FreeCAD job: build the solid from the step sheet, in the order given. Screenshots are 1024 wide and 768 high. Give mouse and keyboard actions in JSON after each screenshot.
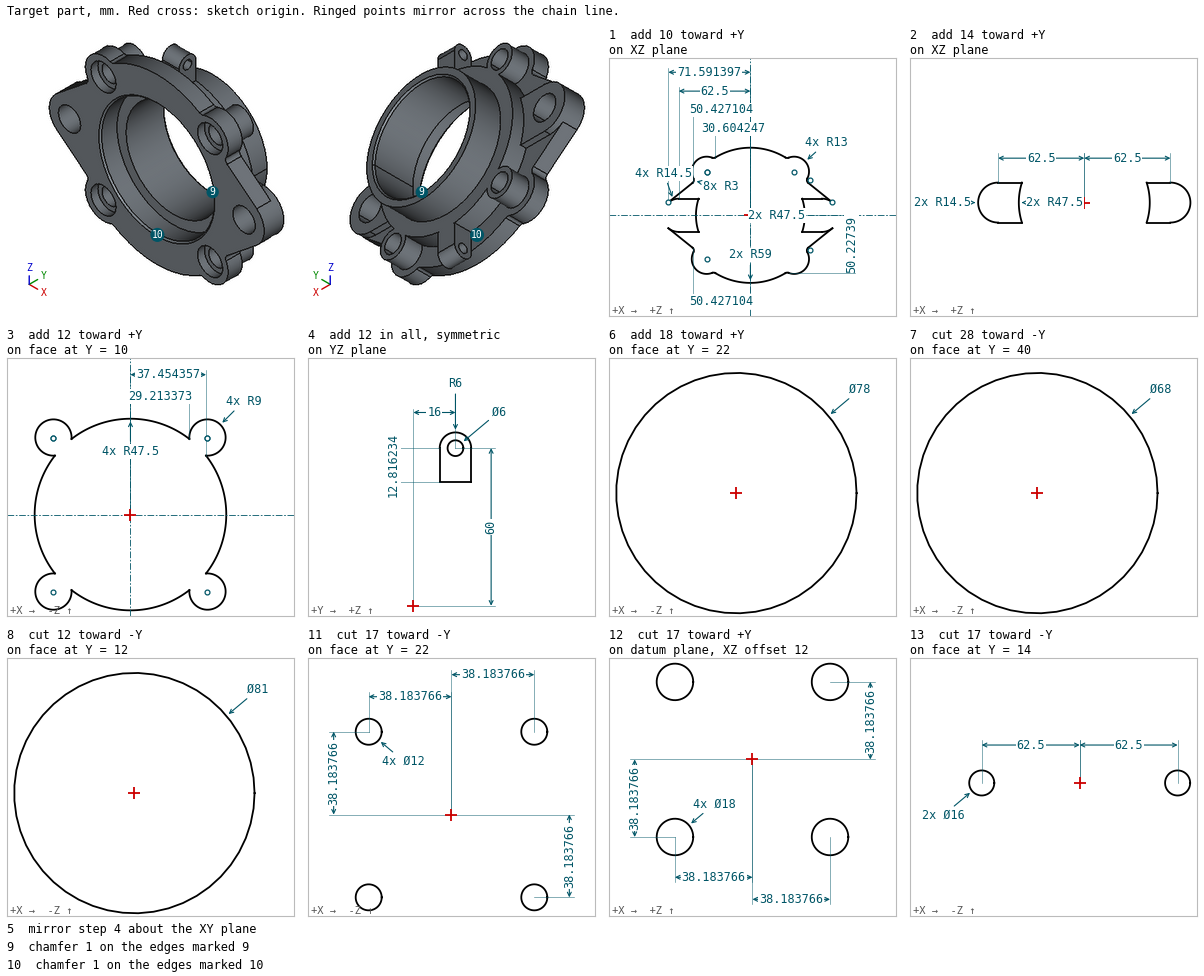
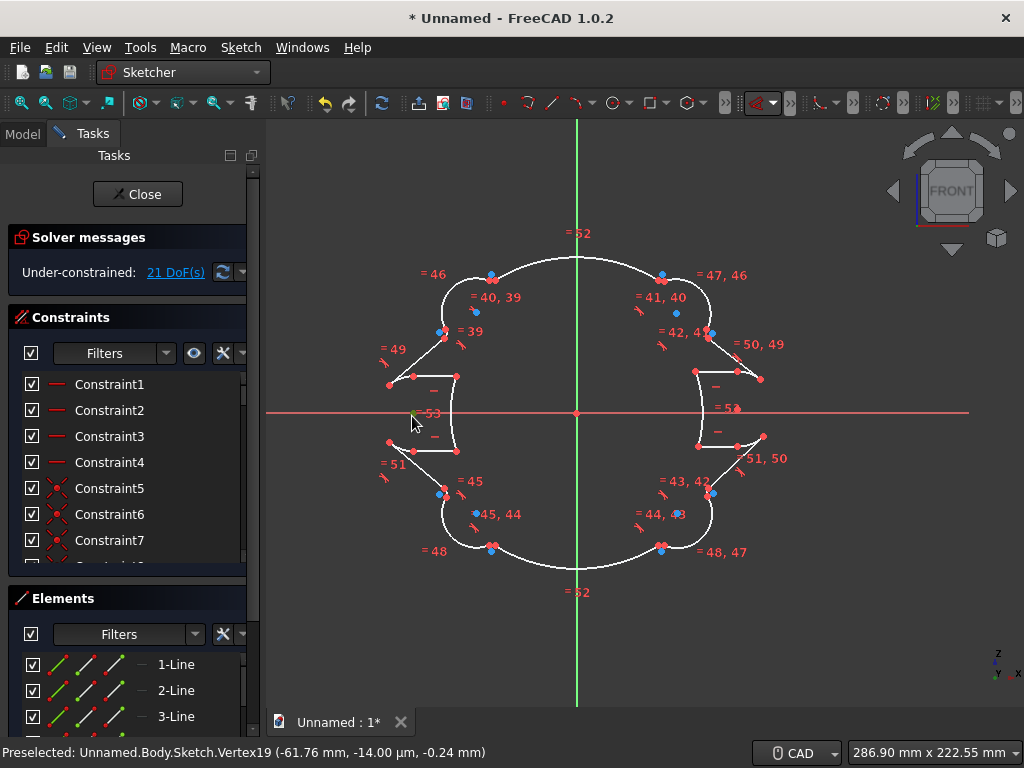
{"action": "left_click", "coordinate": [334, 413]}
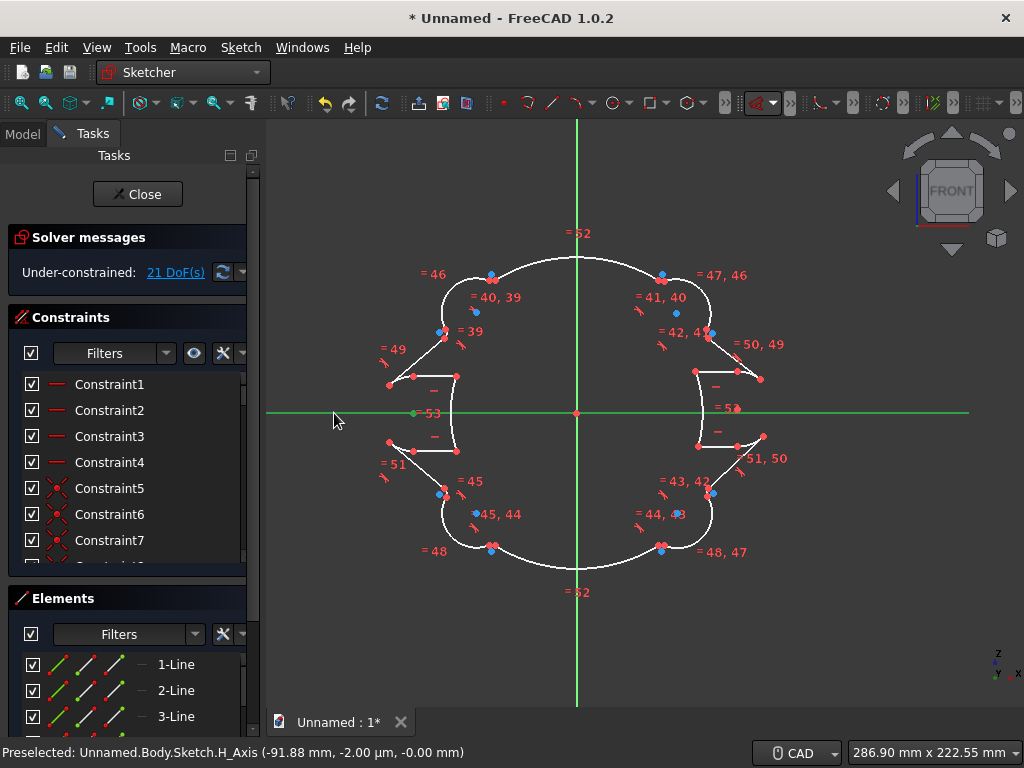
{"action": "key", "text": "c"}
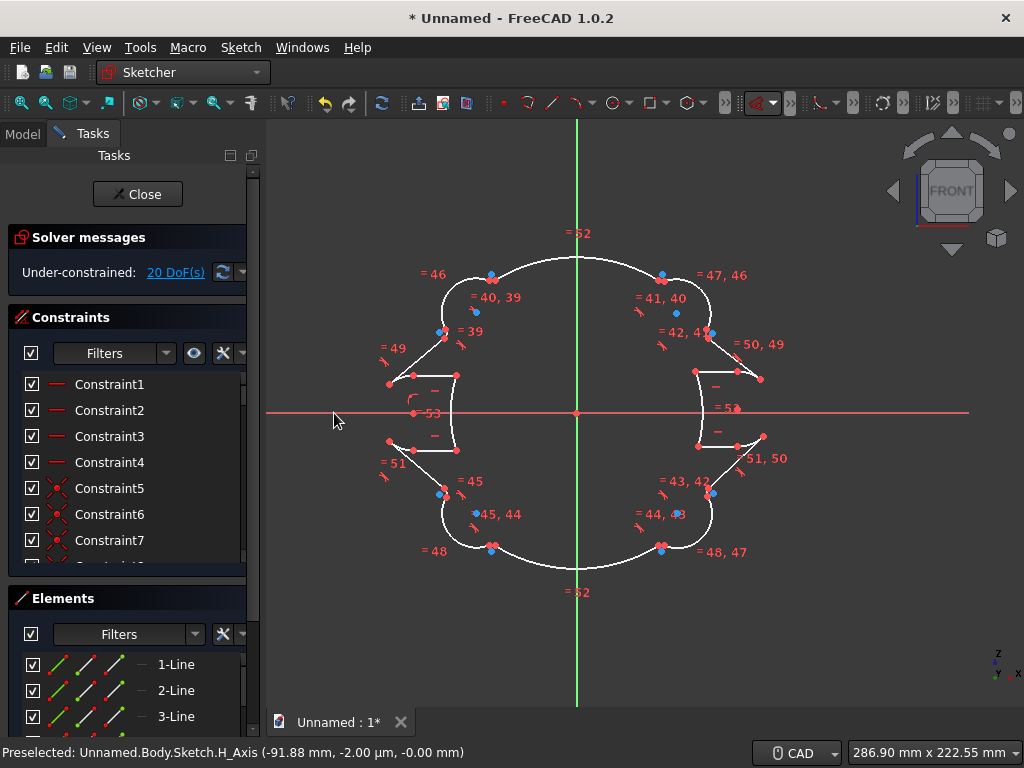
{"action": "left_click", "coordinate": [738, 409]}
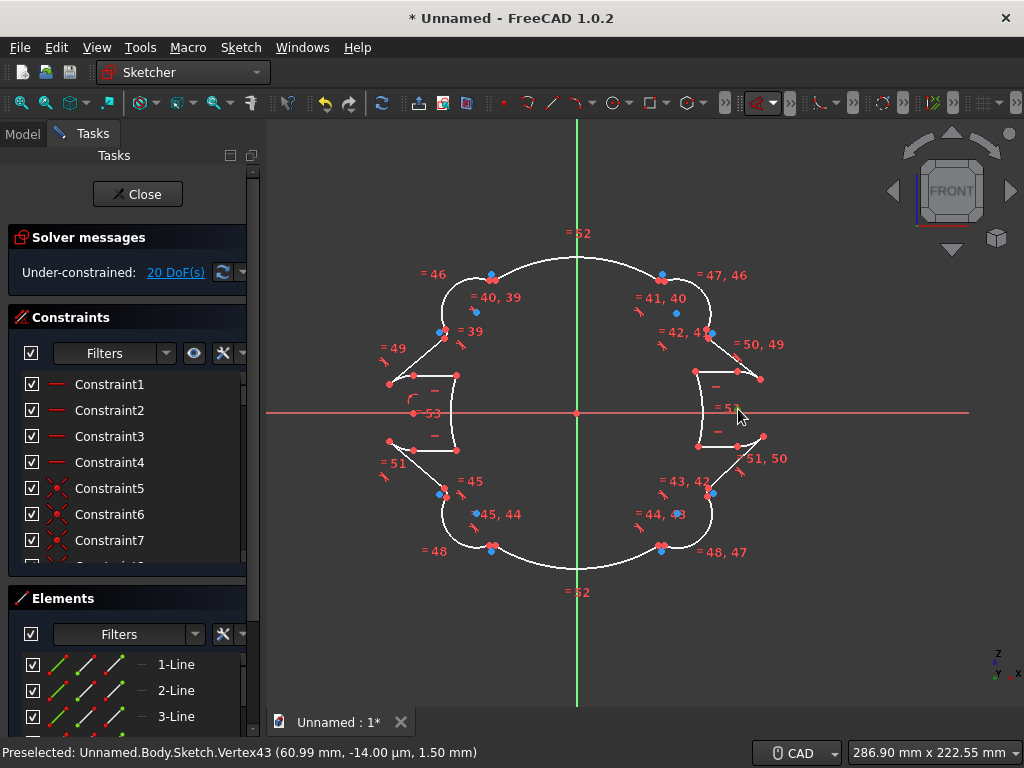
{"action": "left_click", "coordinate": [334, 413]}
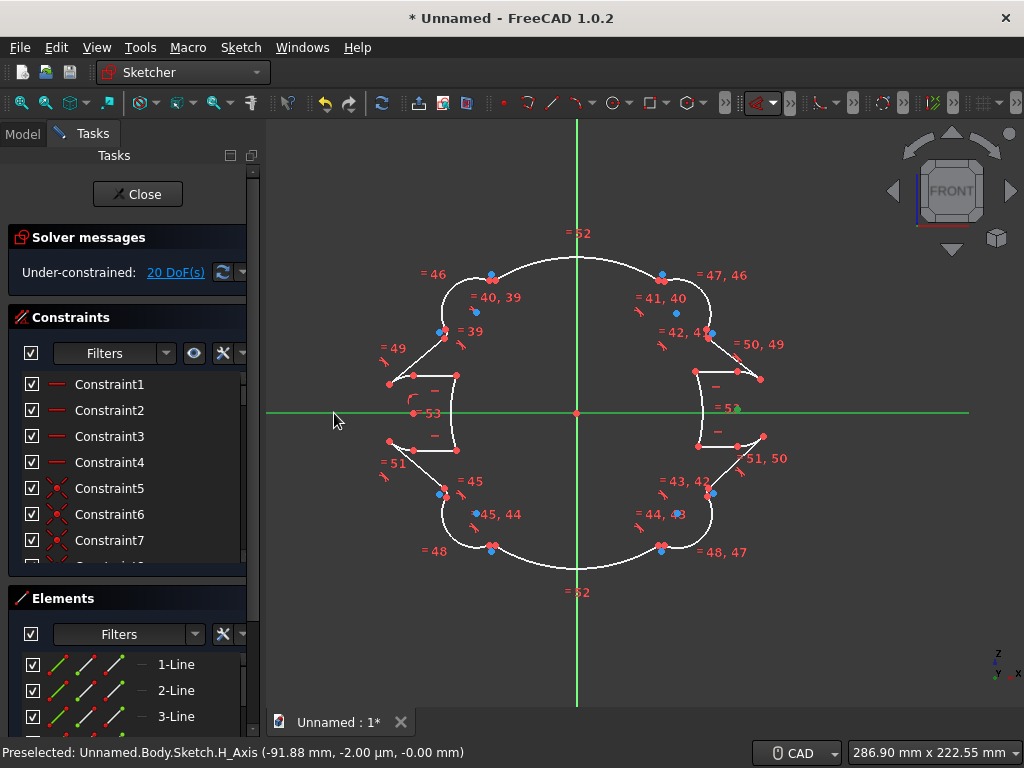
{"action": "key", "text": "c"}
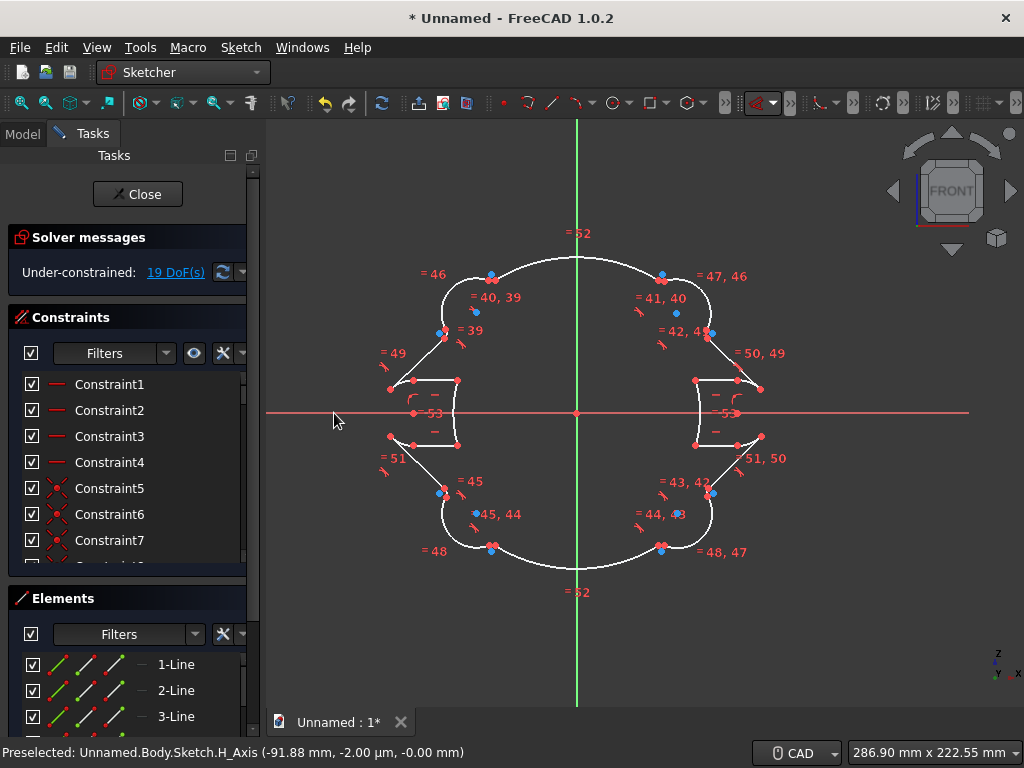
{"action": "left_click", "coordinate": [476, 313]}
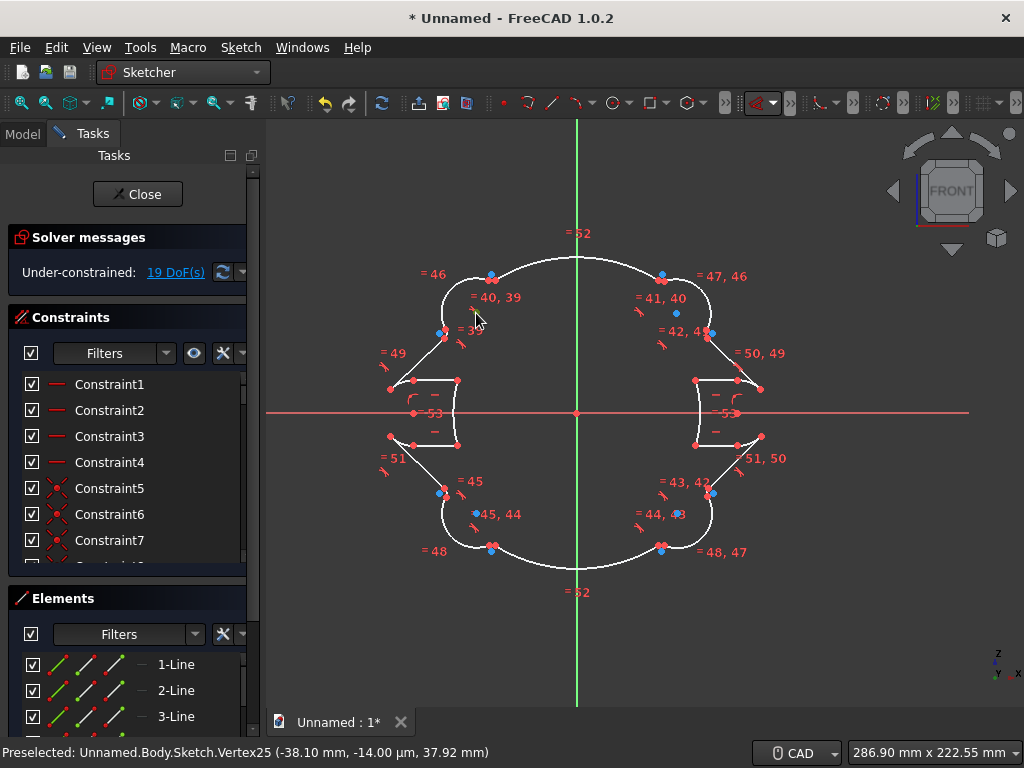
{"action": "left_click", "coordinate": [676, 314]}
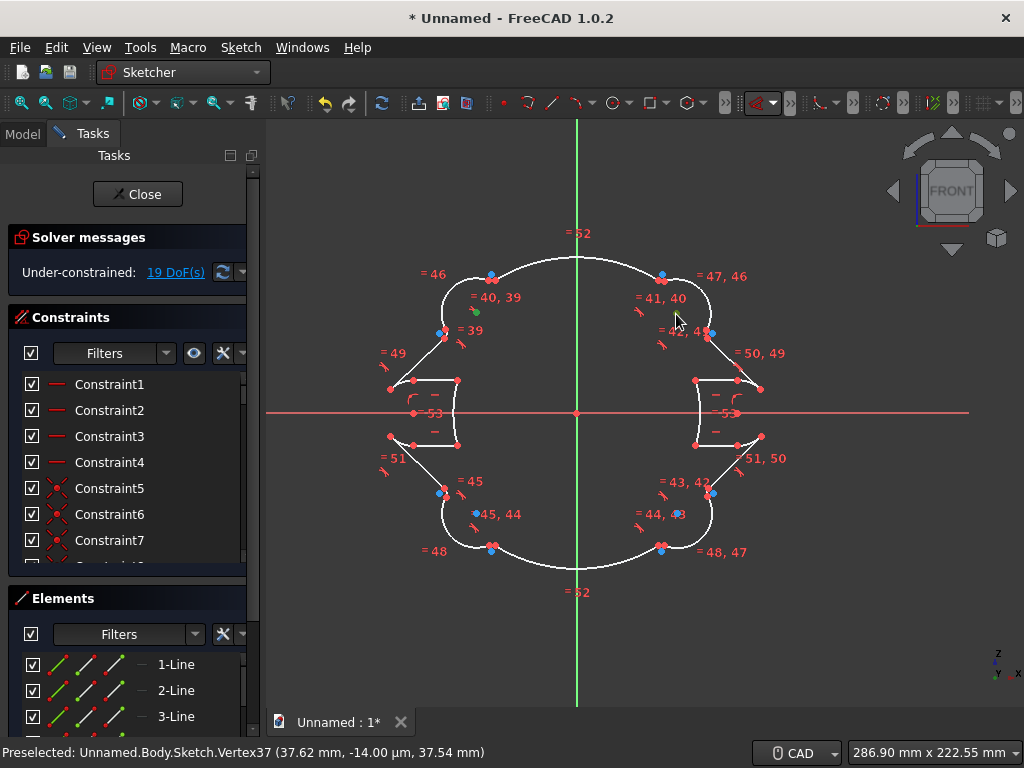
{"action": "left_click", "coordinate": [577, 641]}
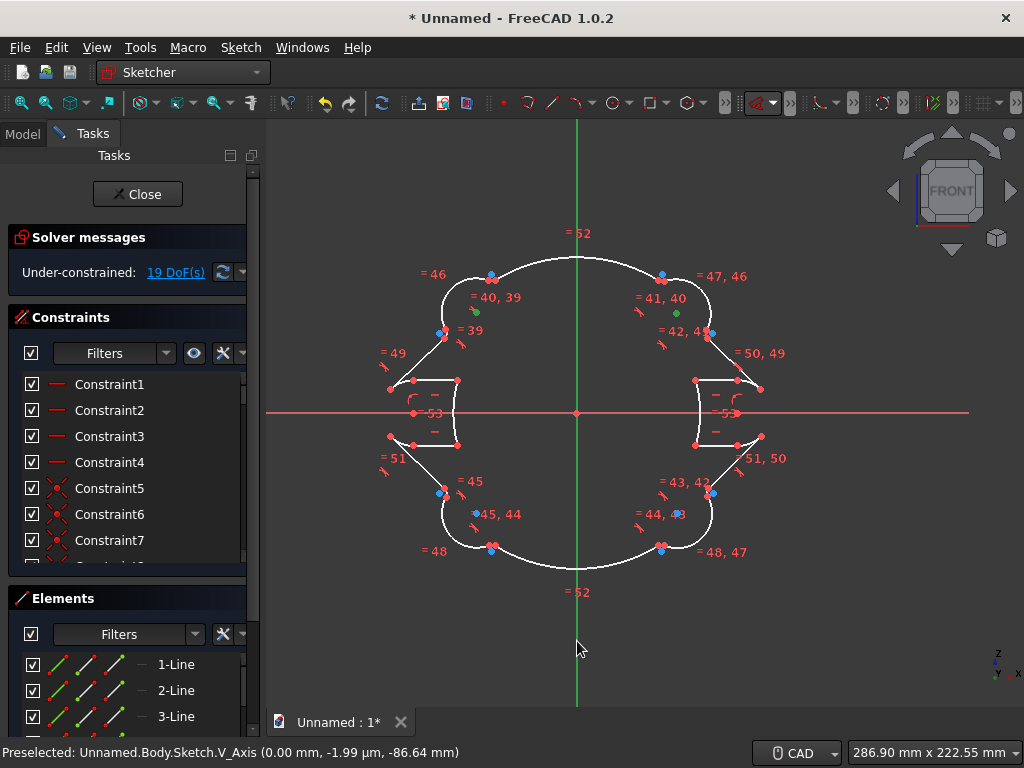
{"action": "key", "text": "s"}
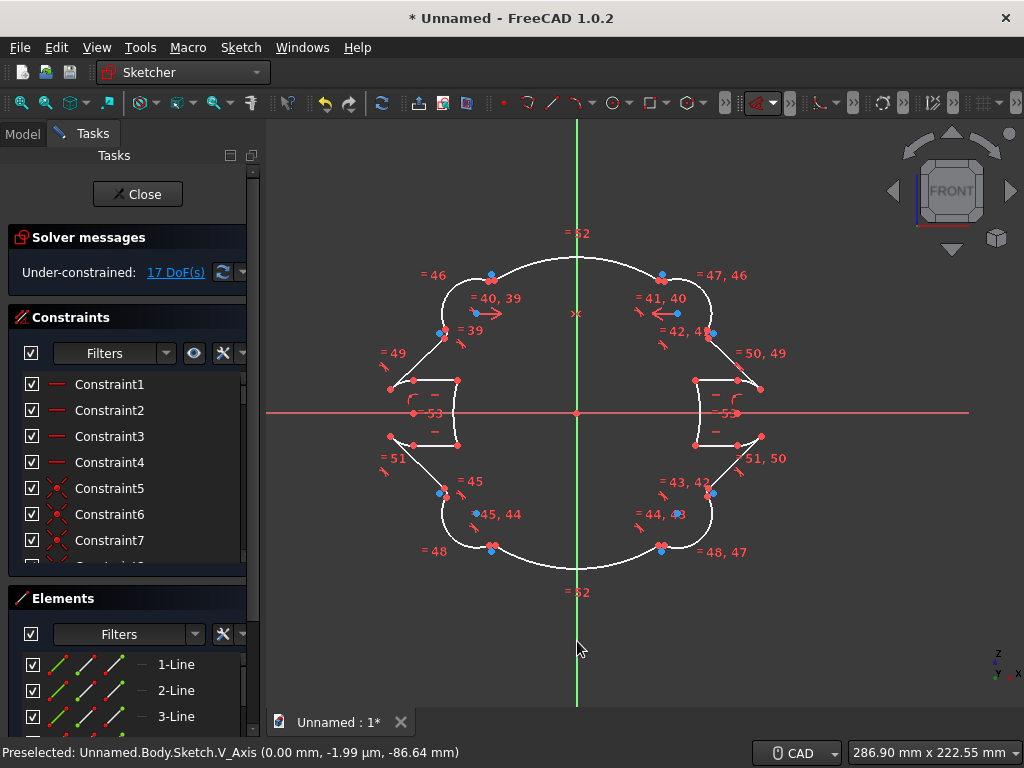
{"action": "scroll", "coordinate": [713, 334], "scroll_direction": "up", "scroll_amount": 3}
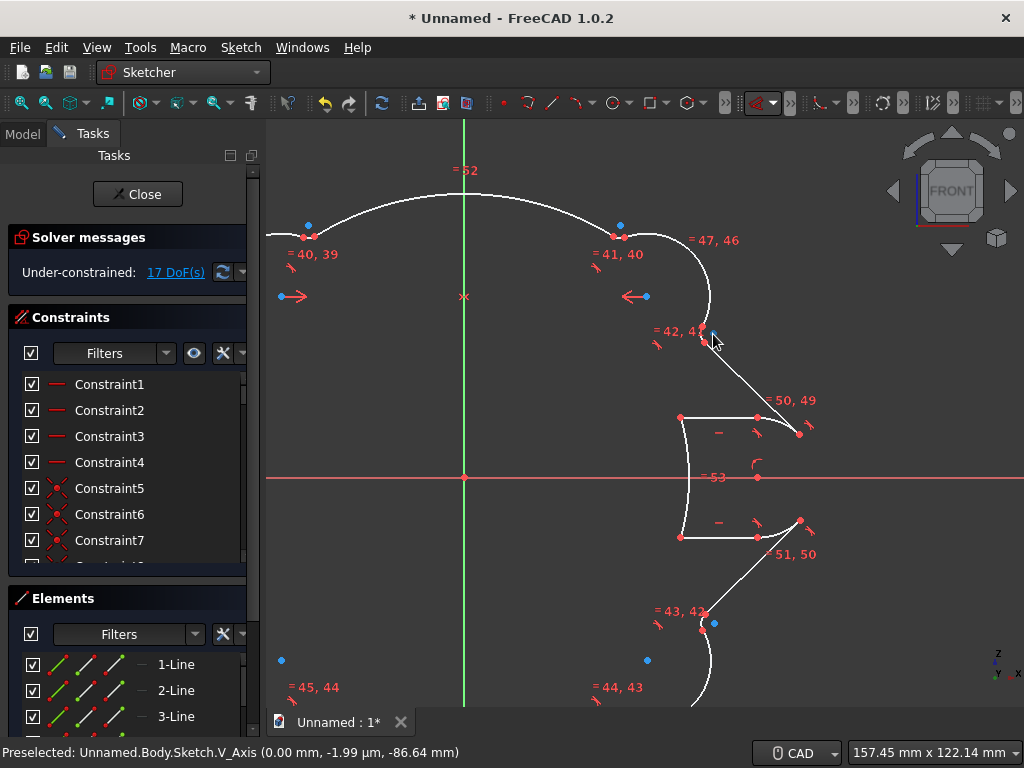
{"action": "left_click", "coordinate": [713, 333]}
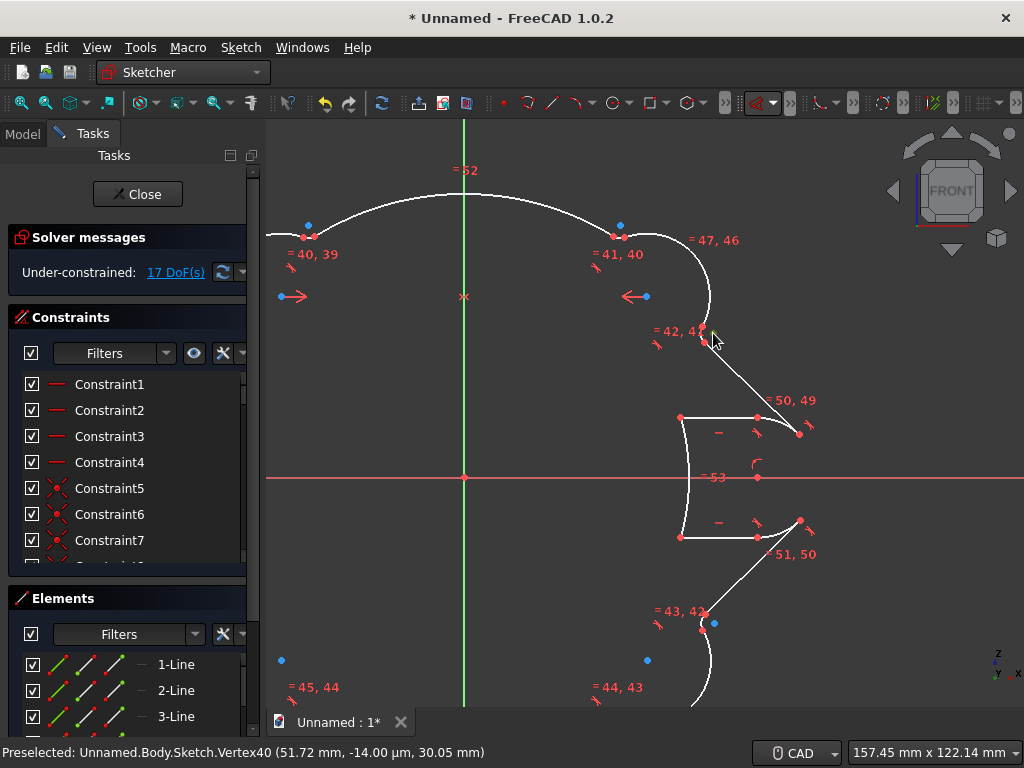
{"action": "left_click", "coordinate": [714, 624]}